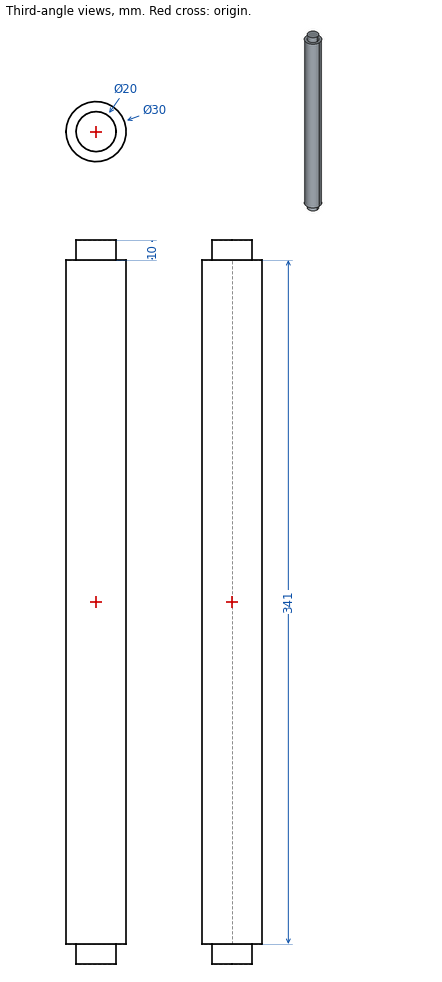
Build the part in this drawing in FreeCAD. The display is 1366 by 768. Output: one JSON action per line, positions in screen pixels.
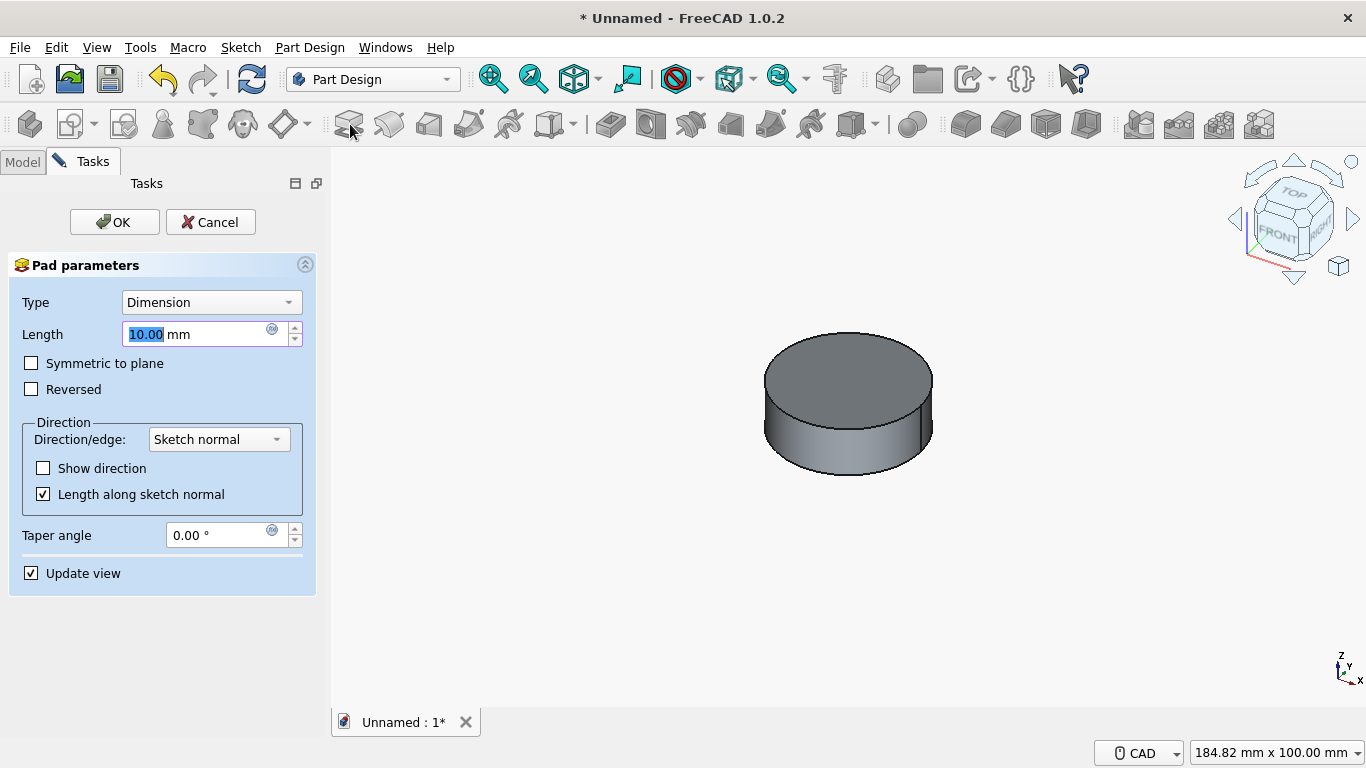
{"action": "type", "text": "341"}
{"action": "key", "text": "Tab"}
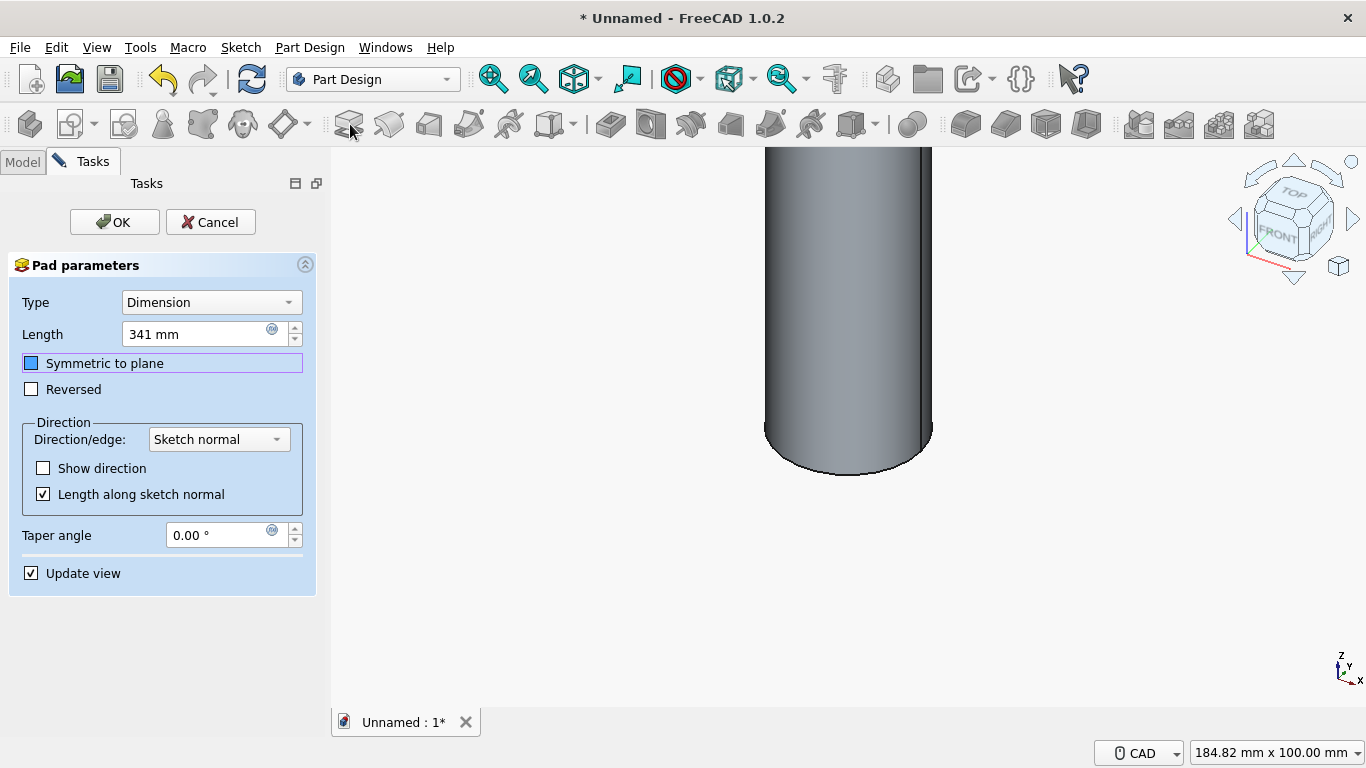
{"action": "left_click", "coordinate": [30, 363]}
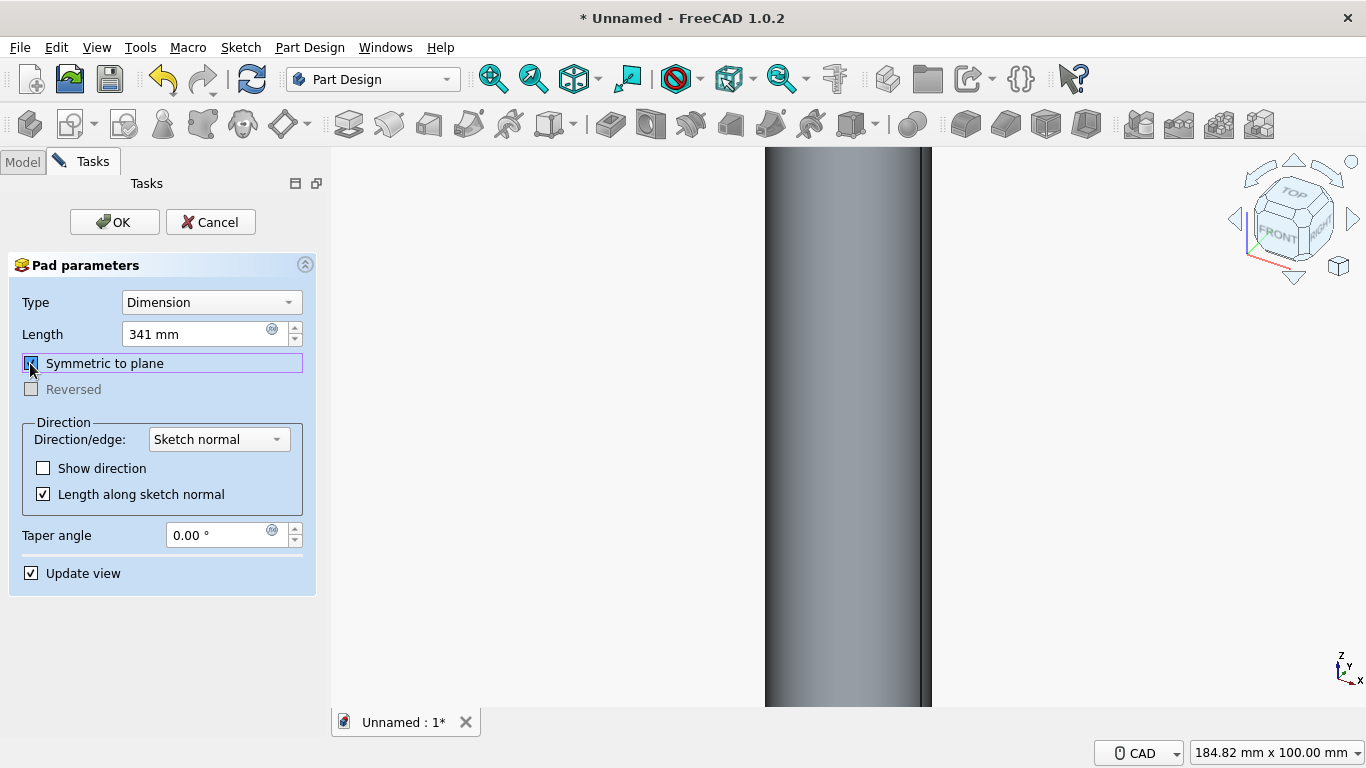
{"action": "left_click", "coordinate": [115, 222]}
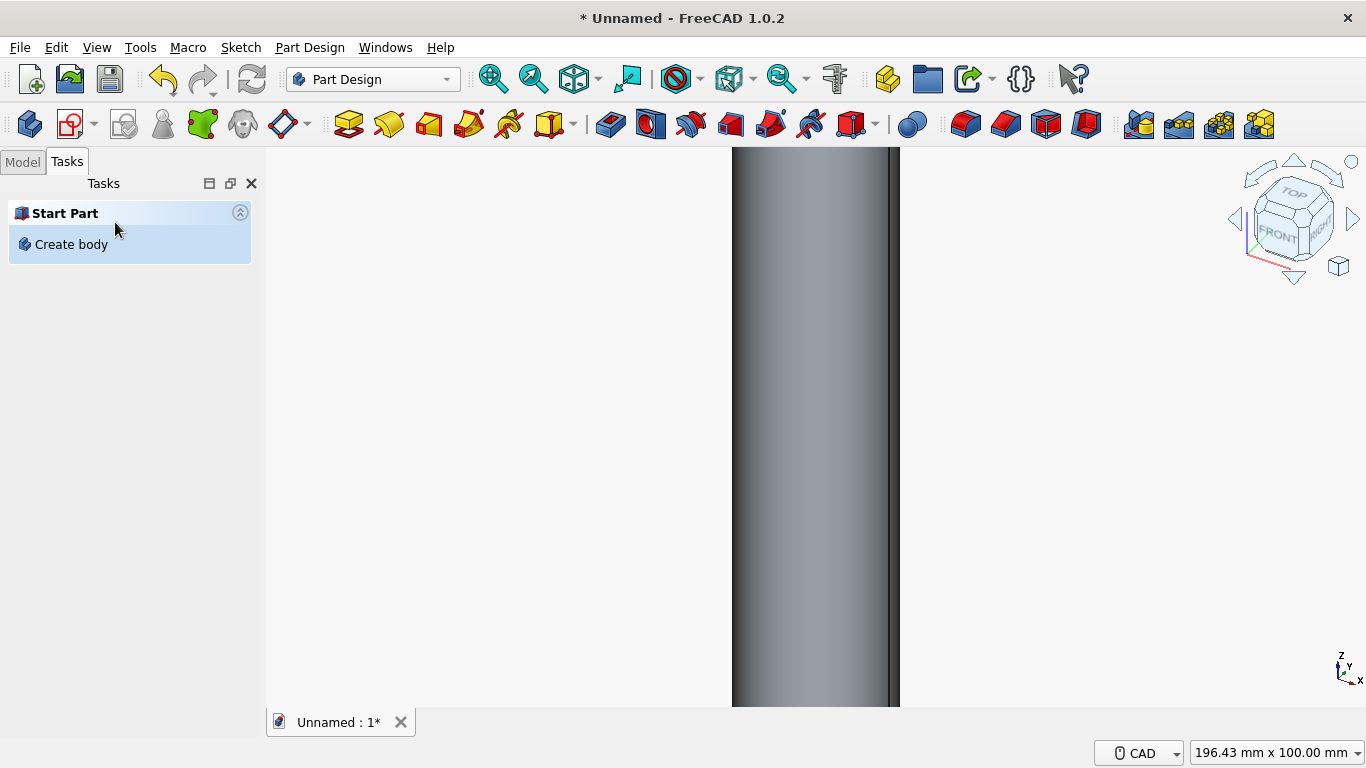
{"action": "left_click", "coordinate": [494, 80]}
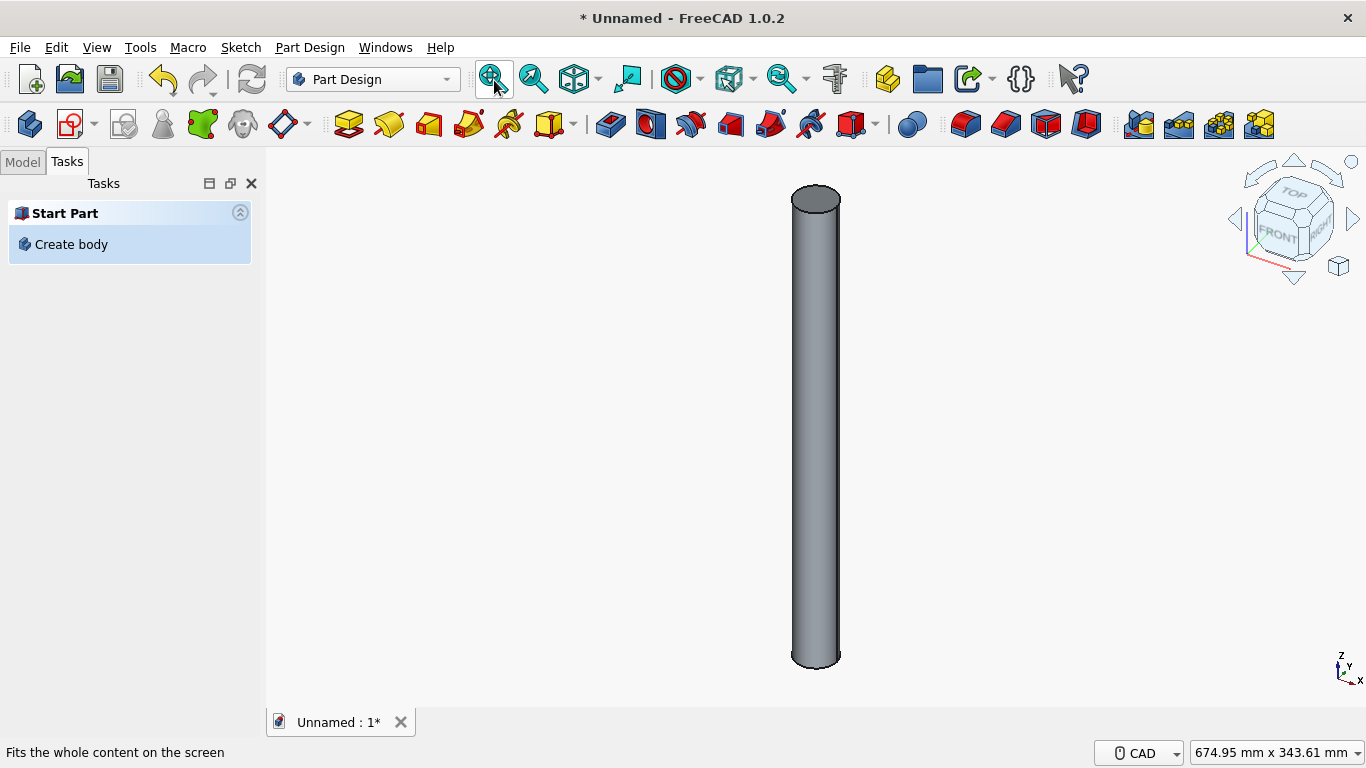
{"action": "left_click", "coordinate": [816, 198]}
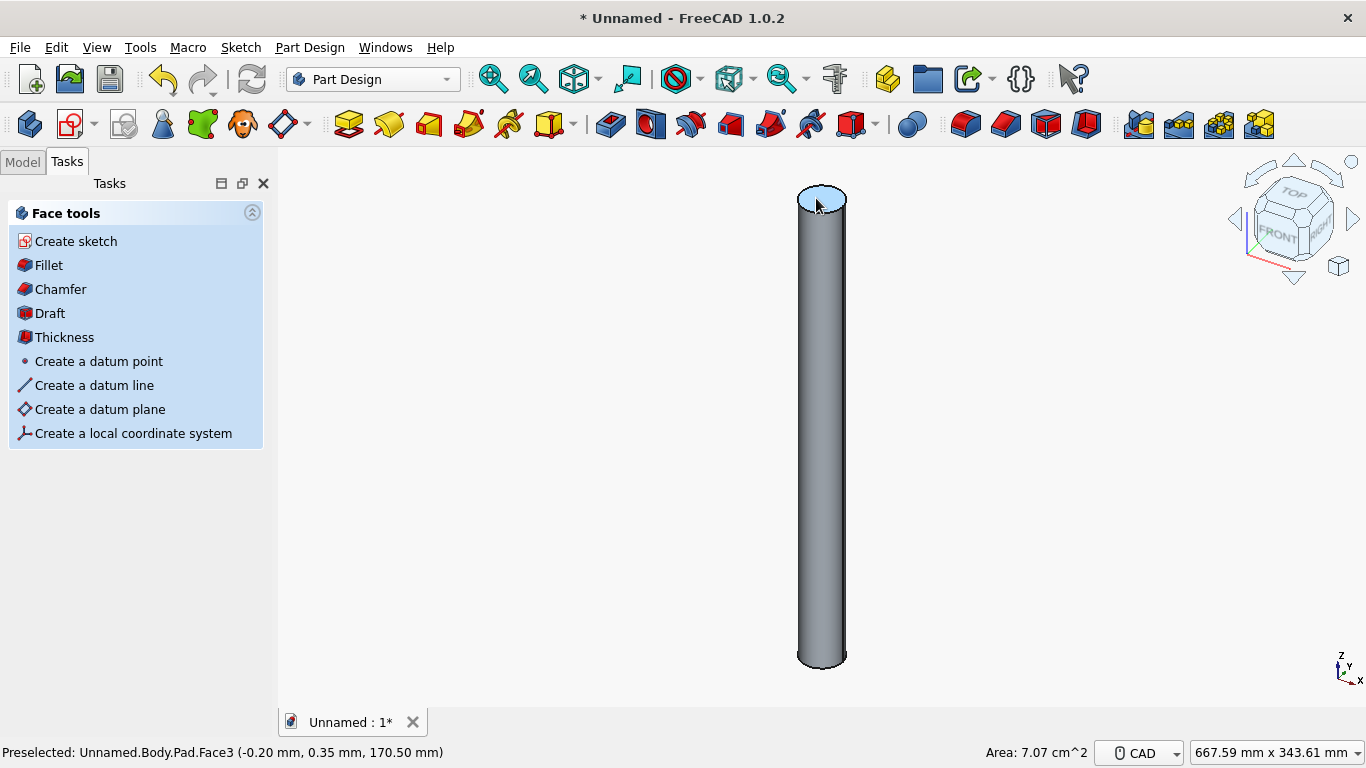
{"action": "left_click", "coordinate": [70, 124]}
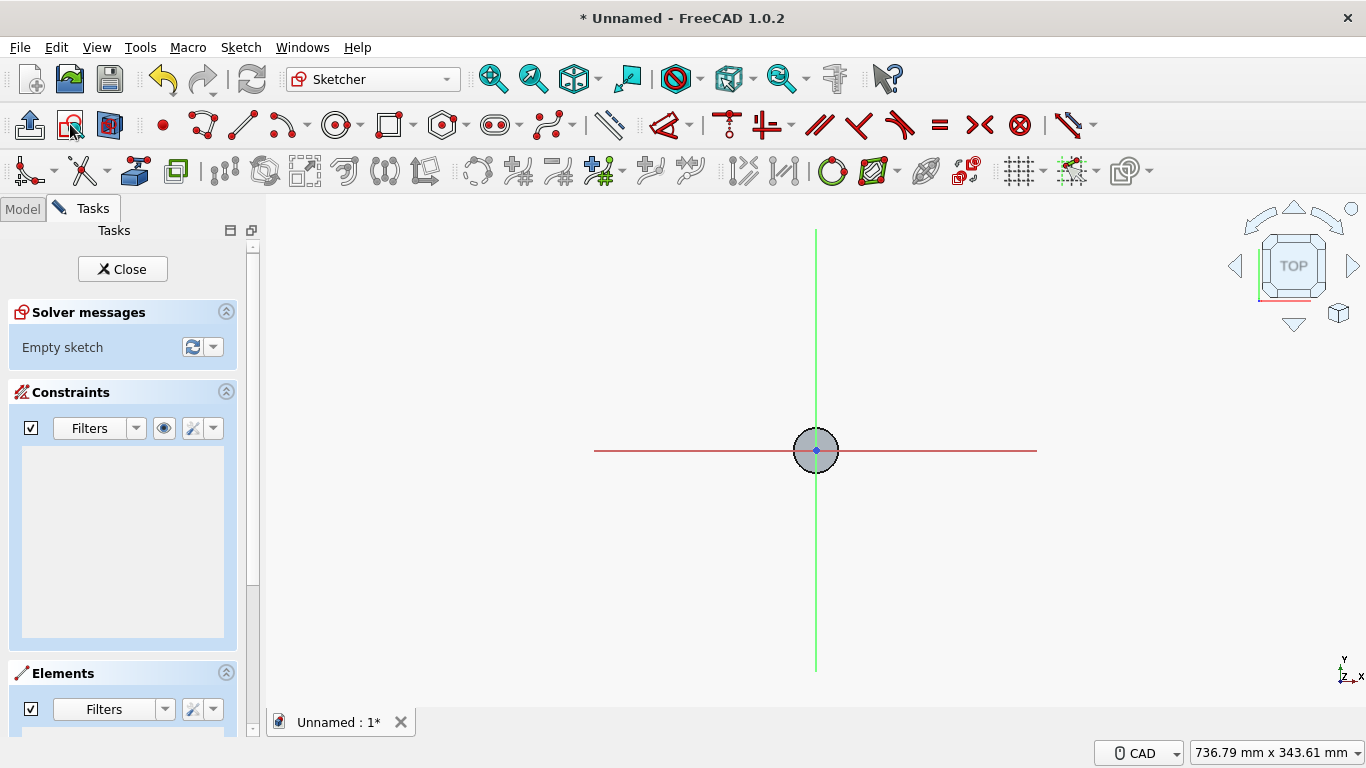
{"action": "scroll", "coordinate": [823, 450], "scroll_direction": "up", "scroll_amount": 12}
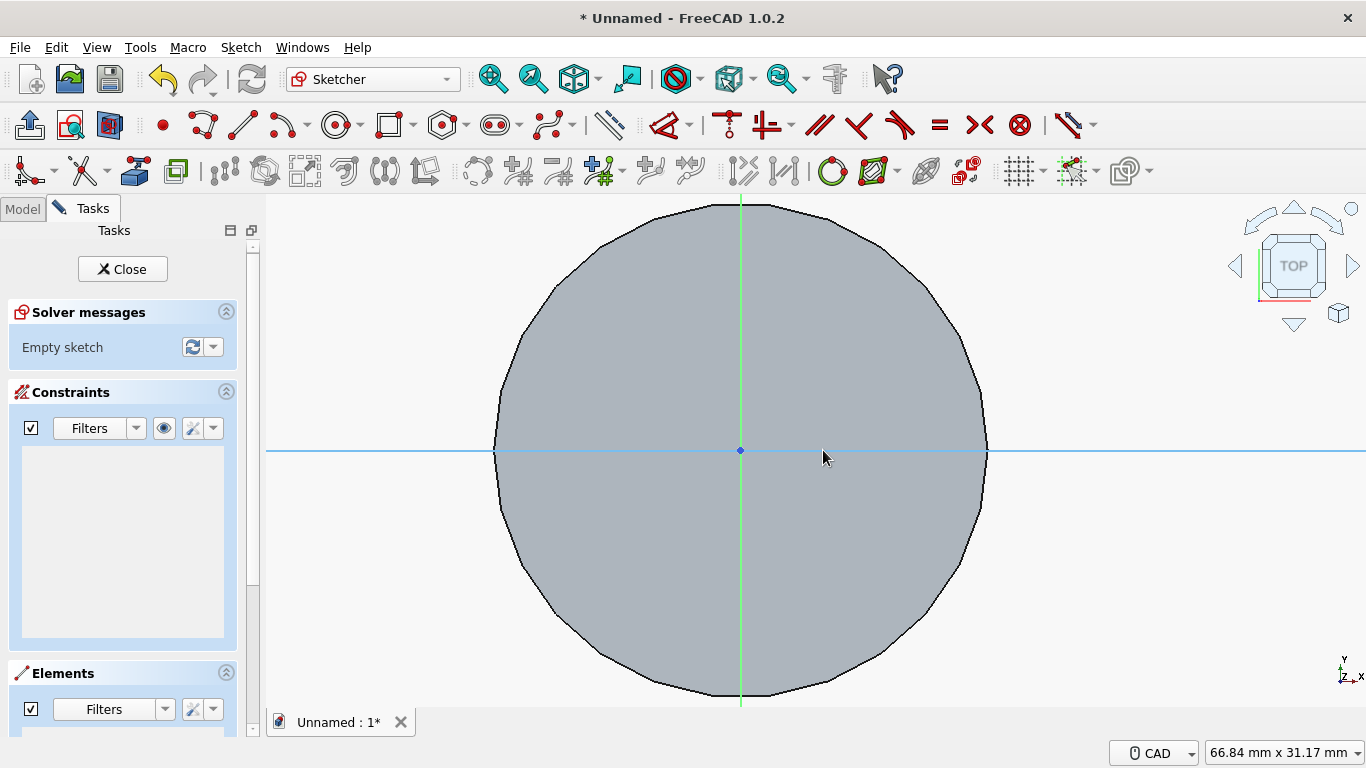
{"action": "left_click", "coordinate": [336, 126]}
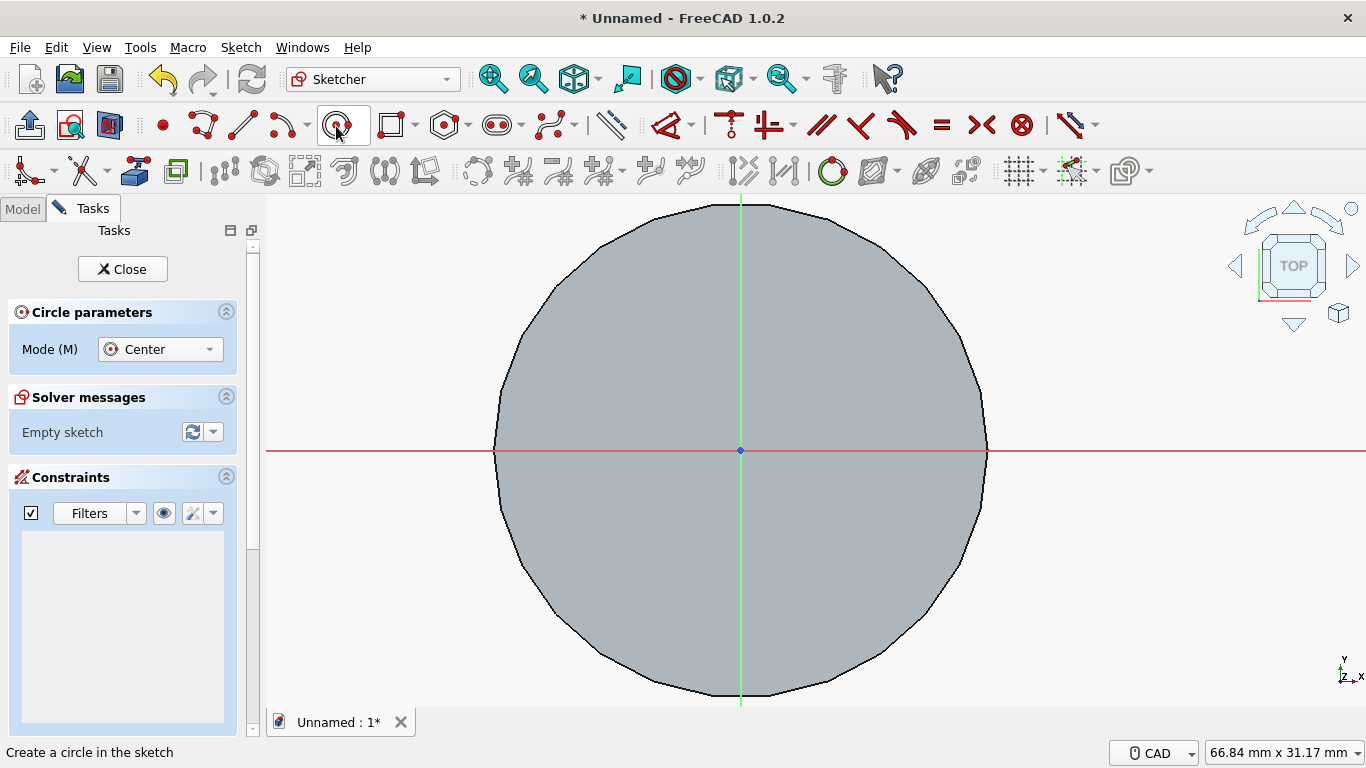
{"action": "left_click", "coordinate": [741, 450]}
{"action": "mouse_move", "coordinate": [857, 334]}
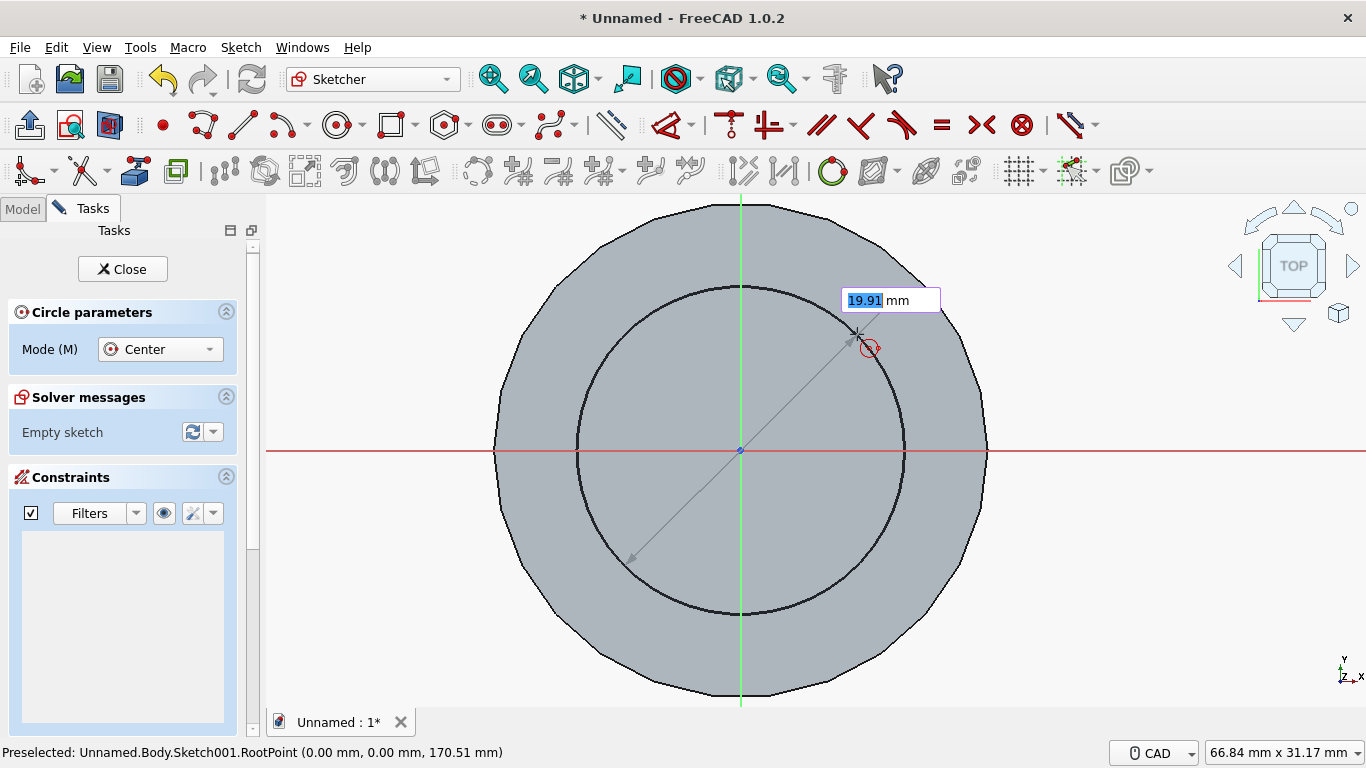
{"action": "type", "text": "20"}
{"action": "key", "text": "Return"}
{"action": "key", "text": "Escape"}